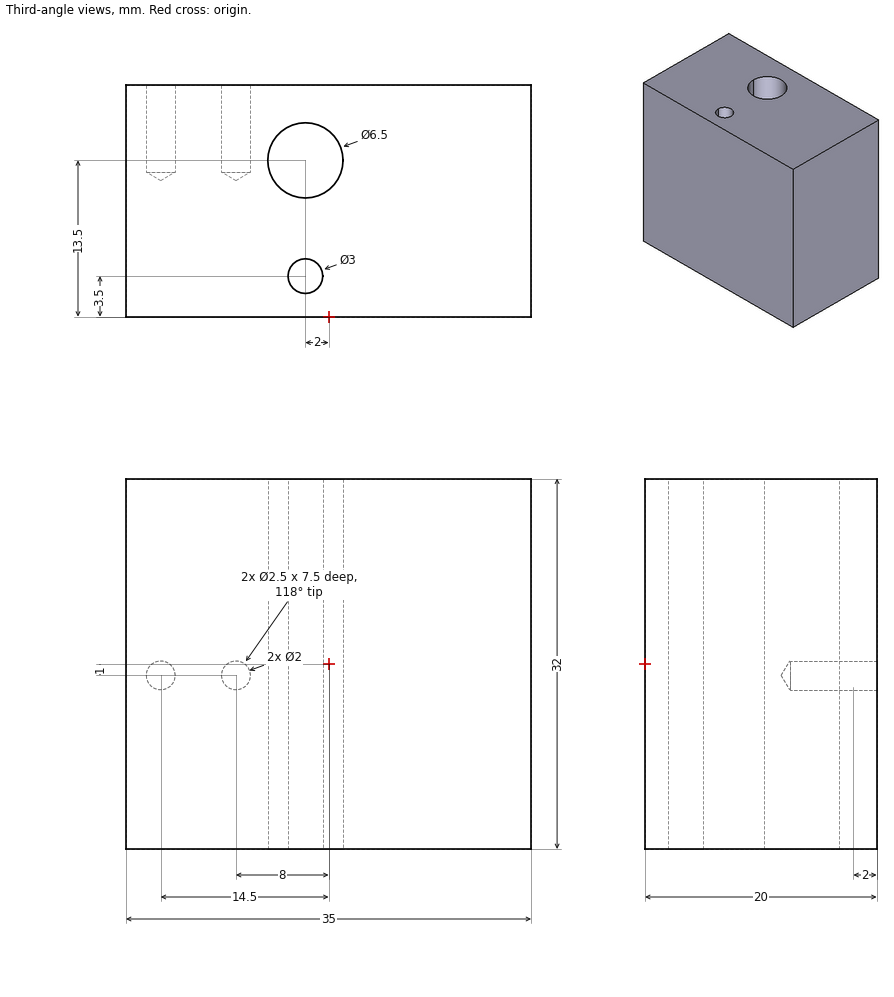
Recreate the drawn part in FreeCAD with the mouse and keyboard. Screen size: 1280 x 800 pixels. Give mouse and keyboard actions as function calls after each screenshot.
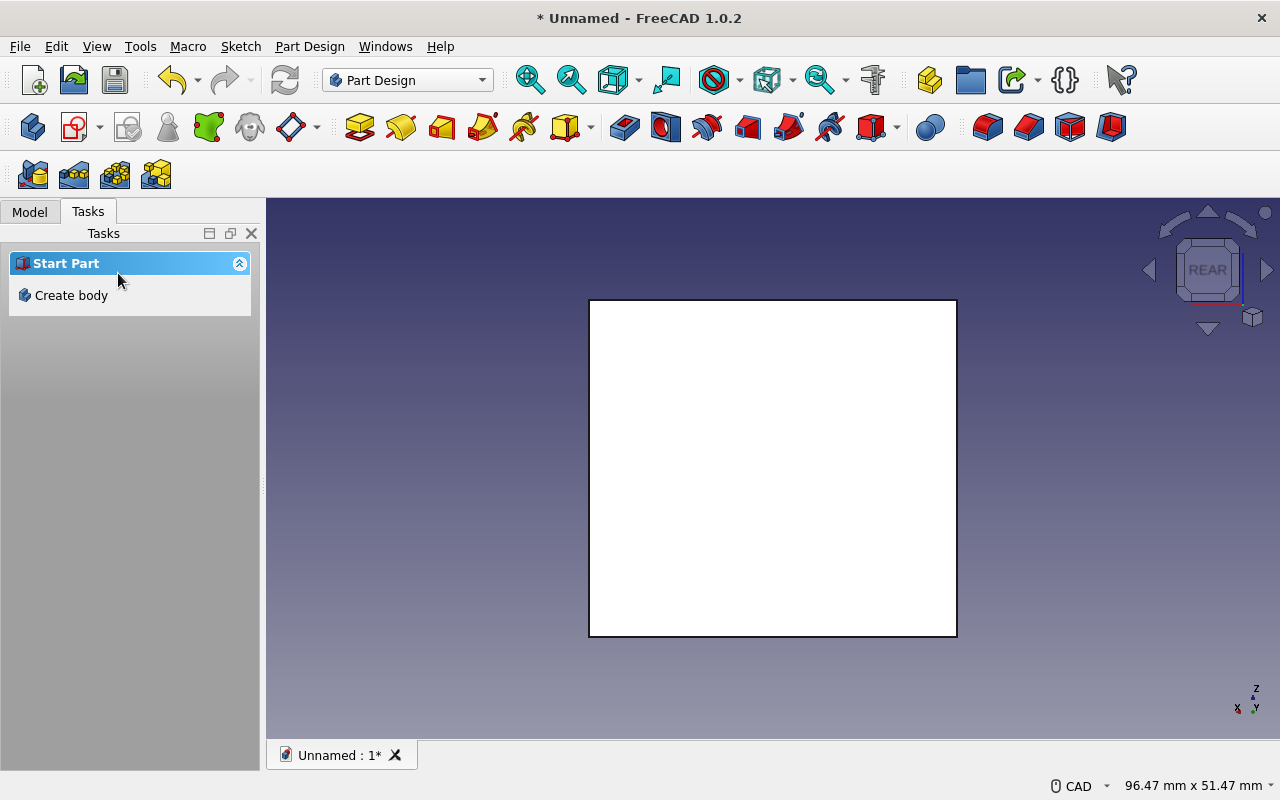
click(773, 468)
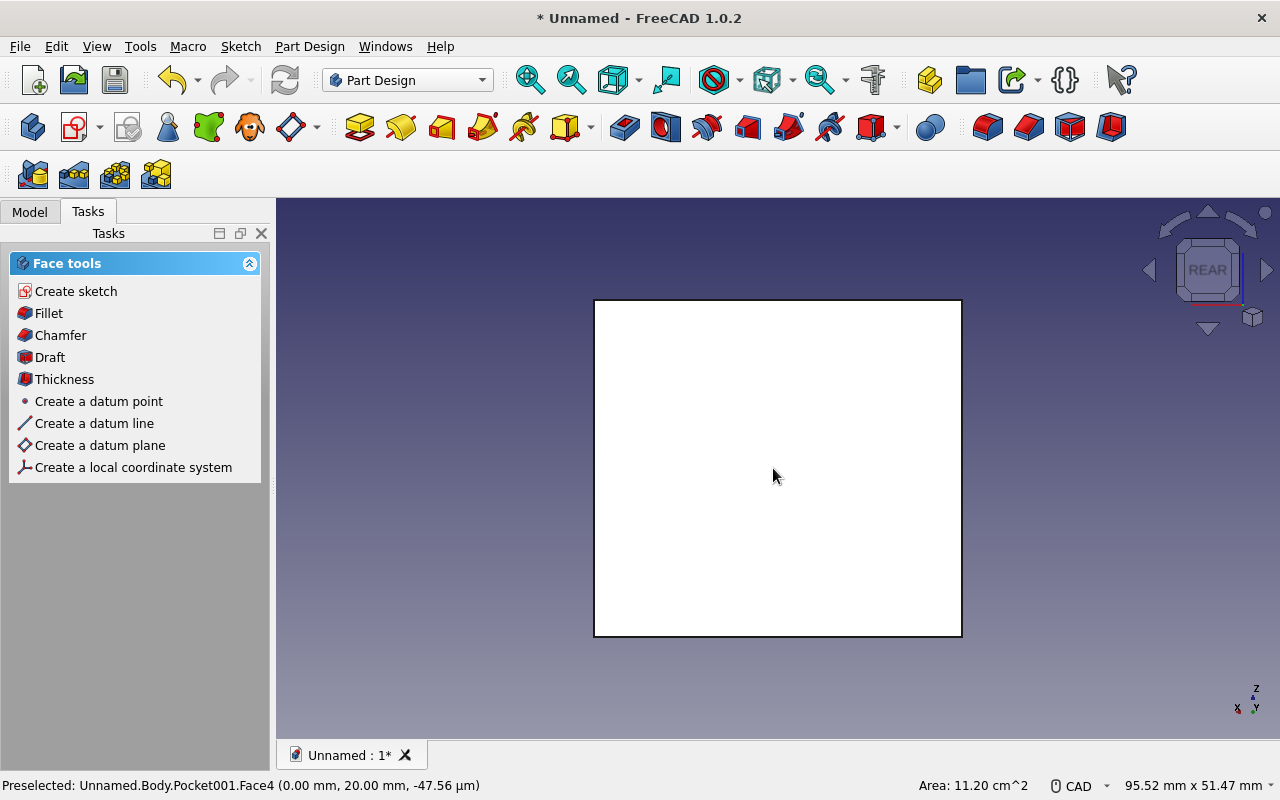
click(74, 128)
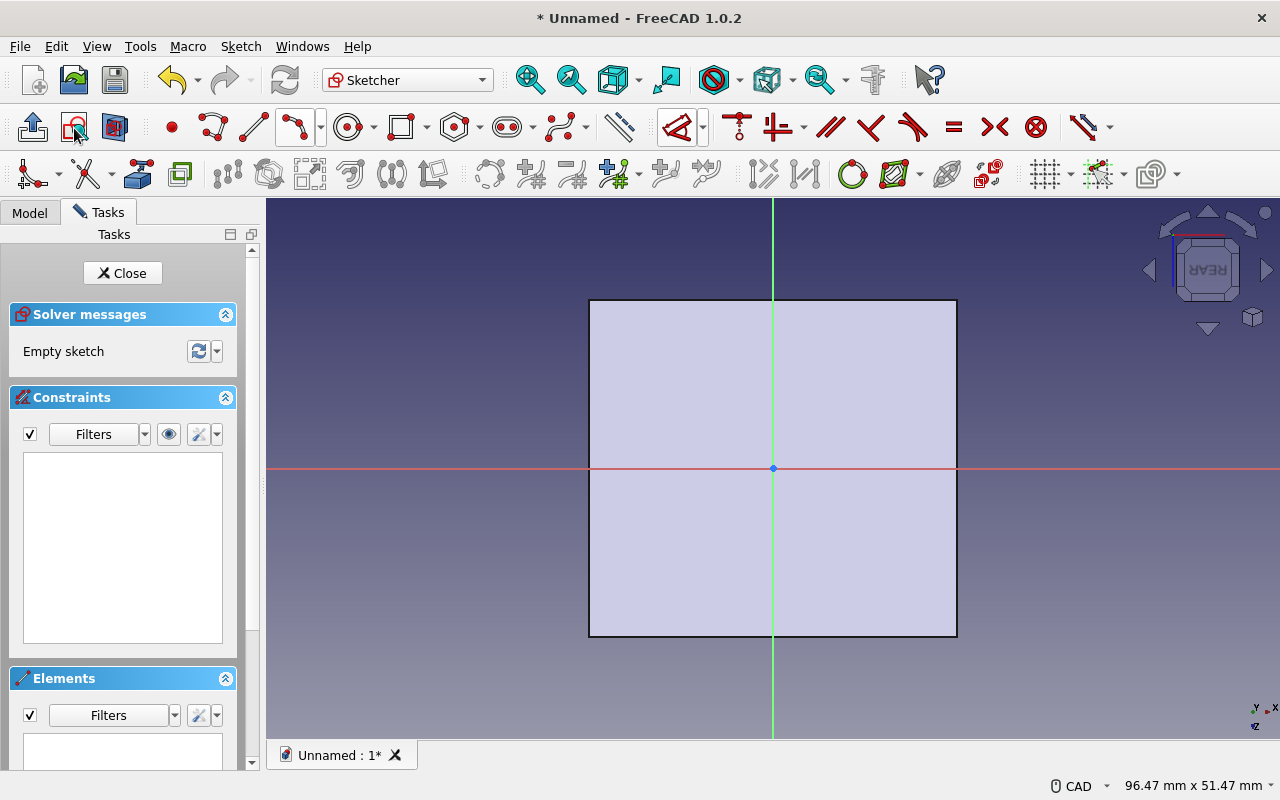
scroll(686, 453, up, 6)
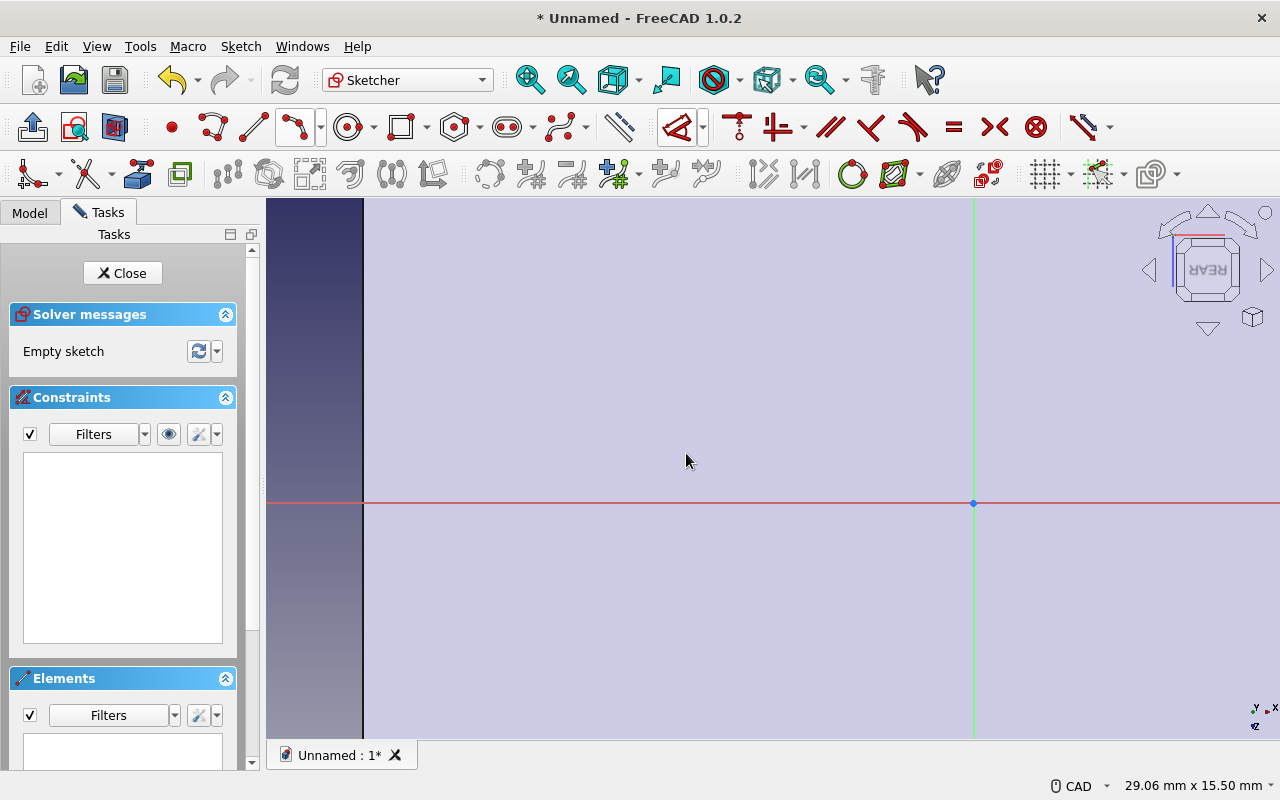
key(g)
key(c)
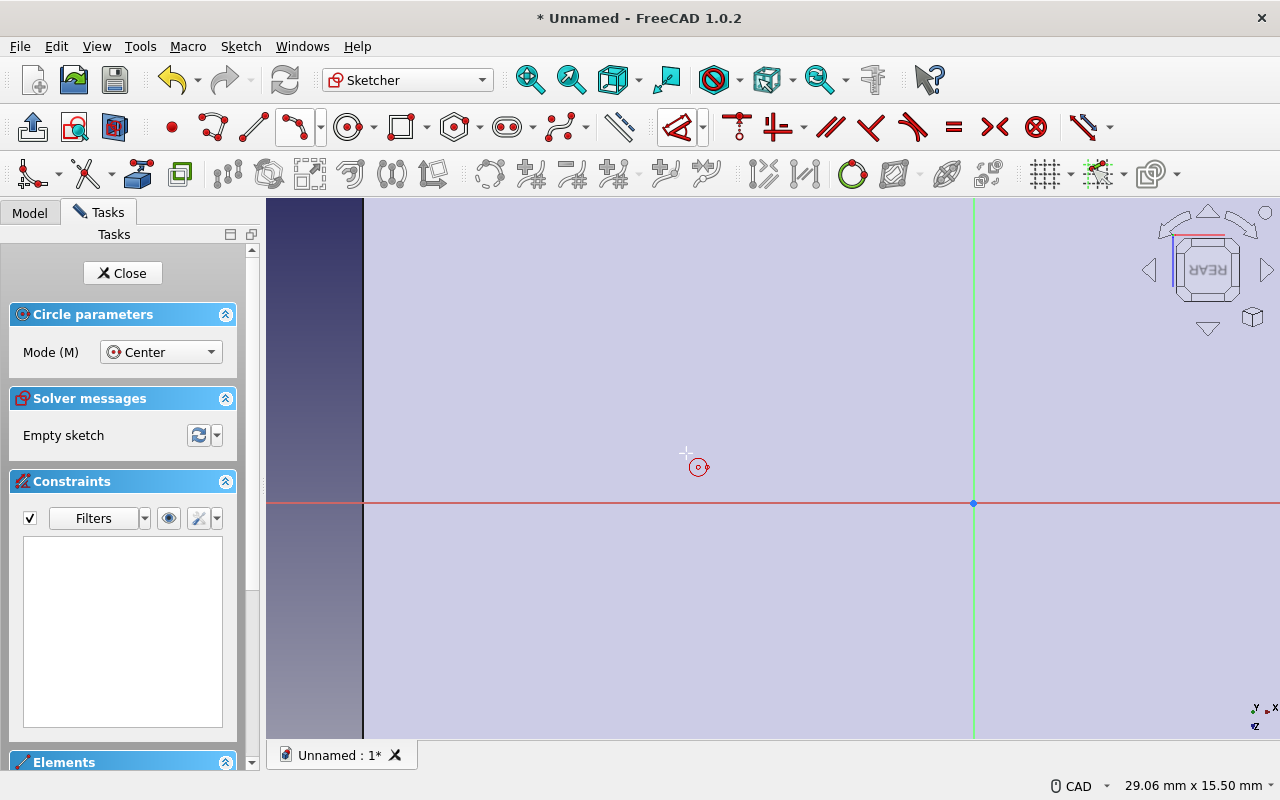
click(695, 468)
click(719, 444)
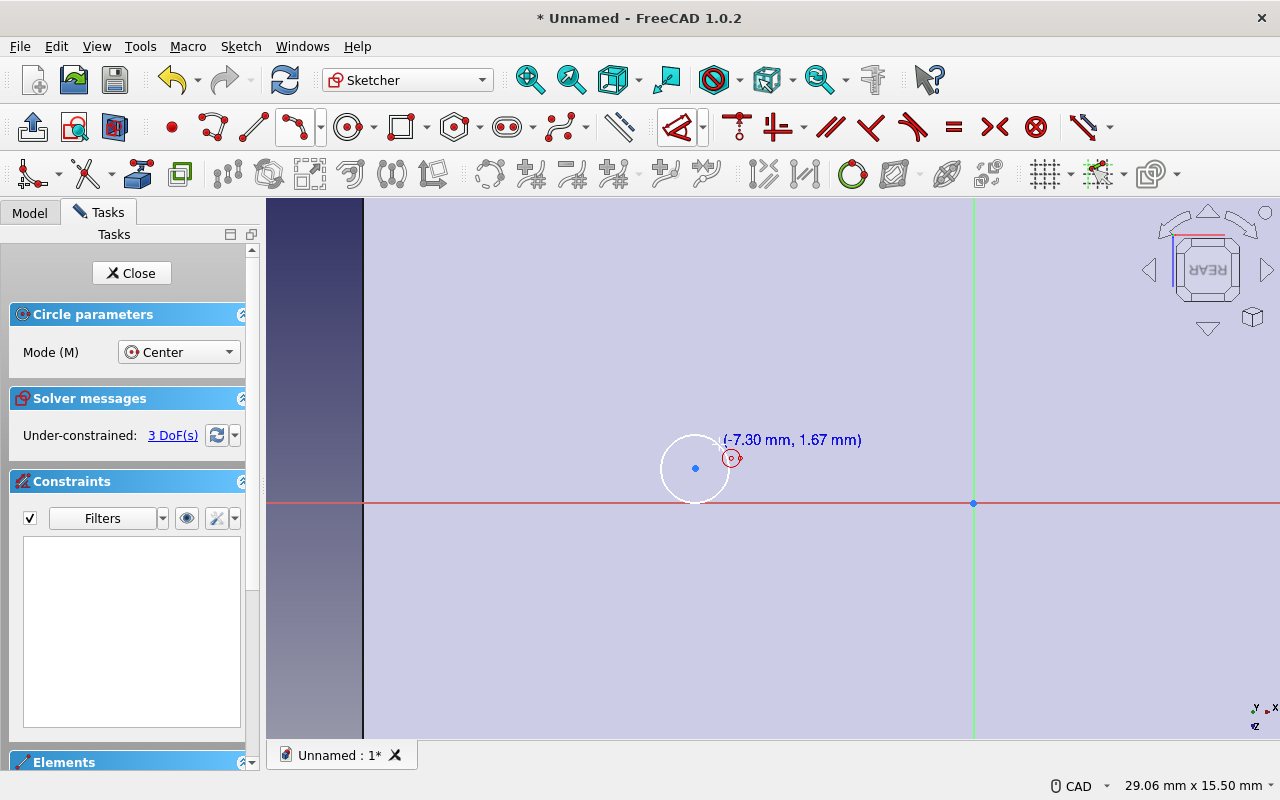
click(468, 468)
click(493, 444)
key(Escape)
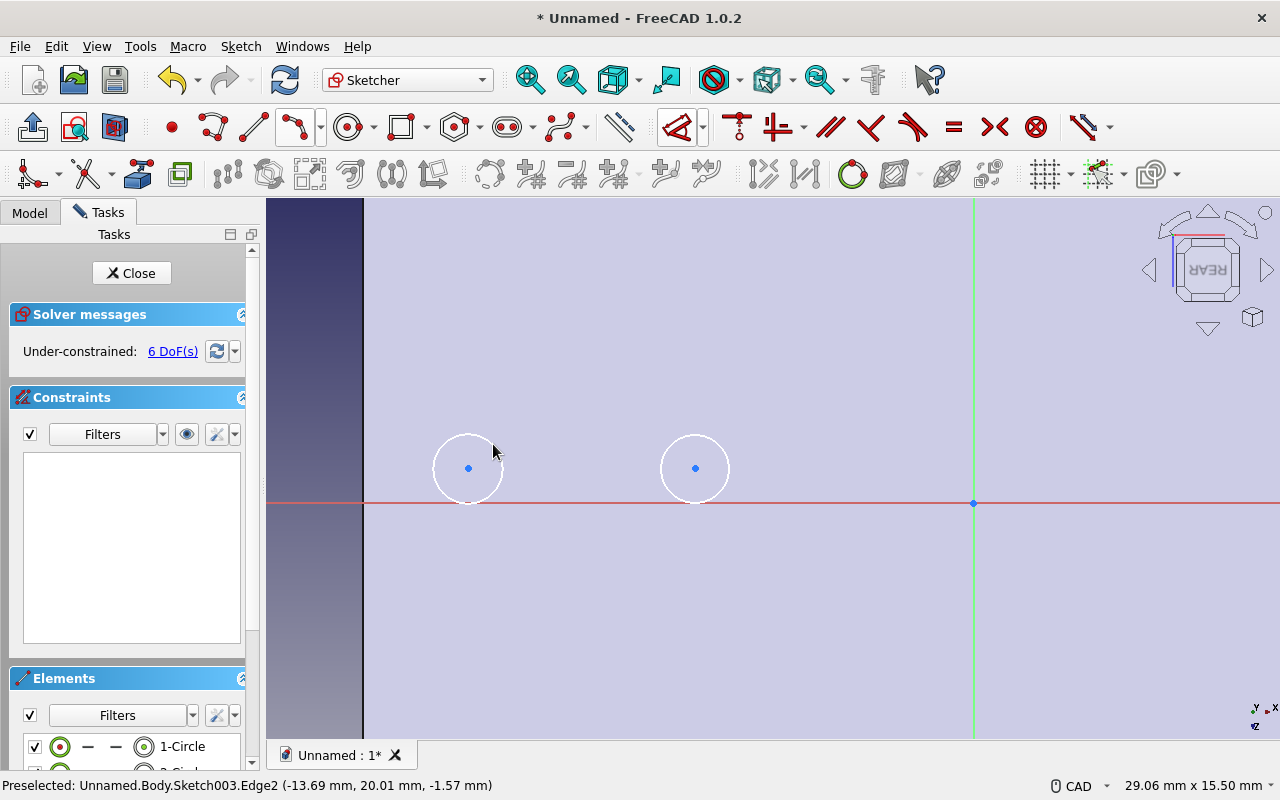
click(719, 445)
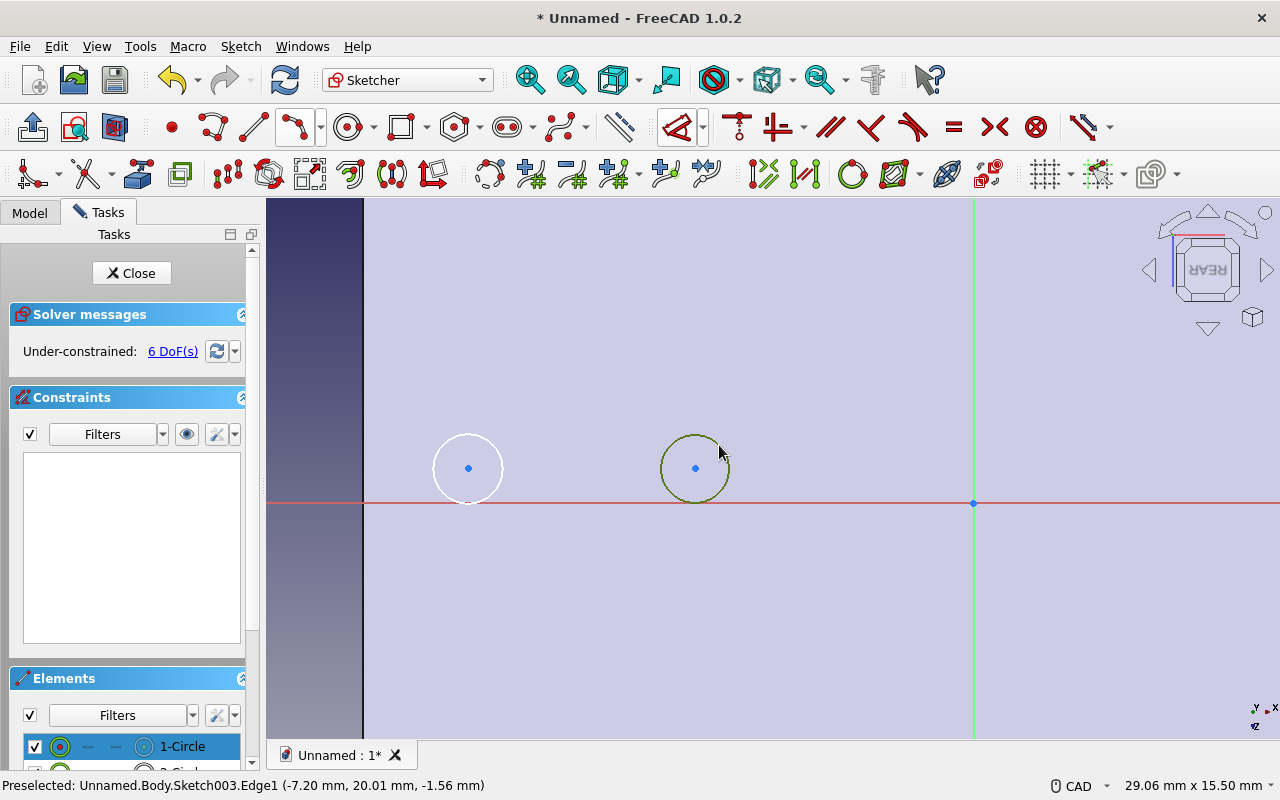
click(492, 444)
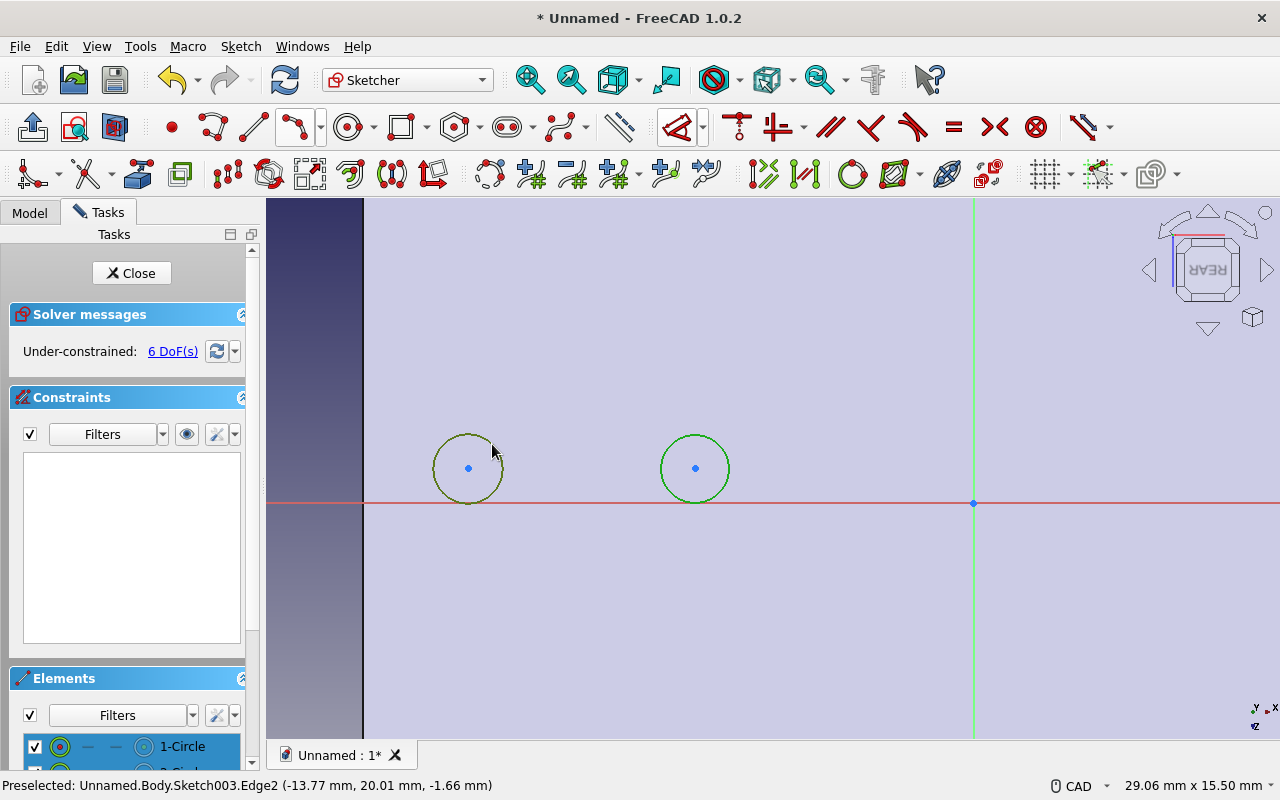
key(e)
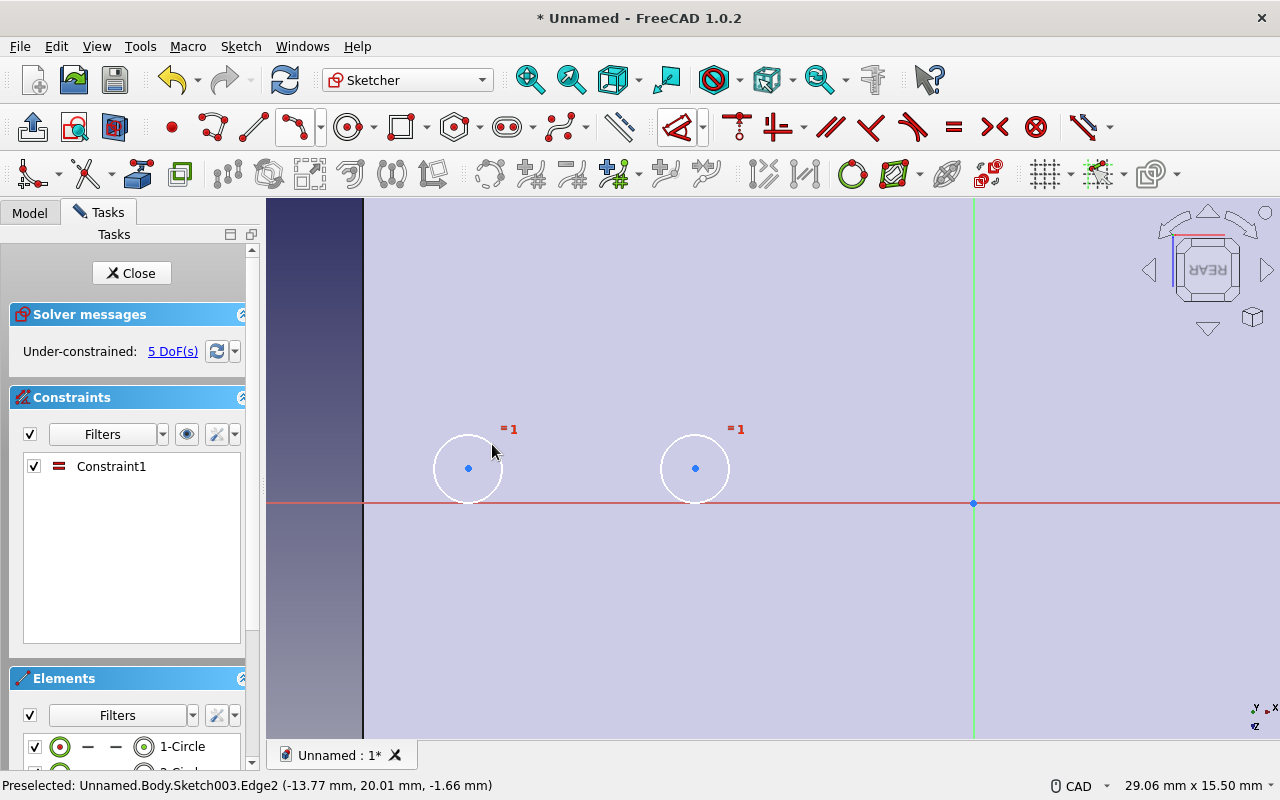
click(719, 445)